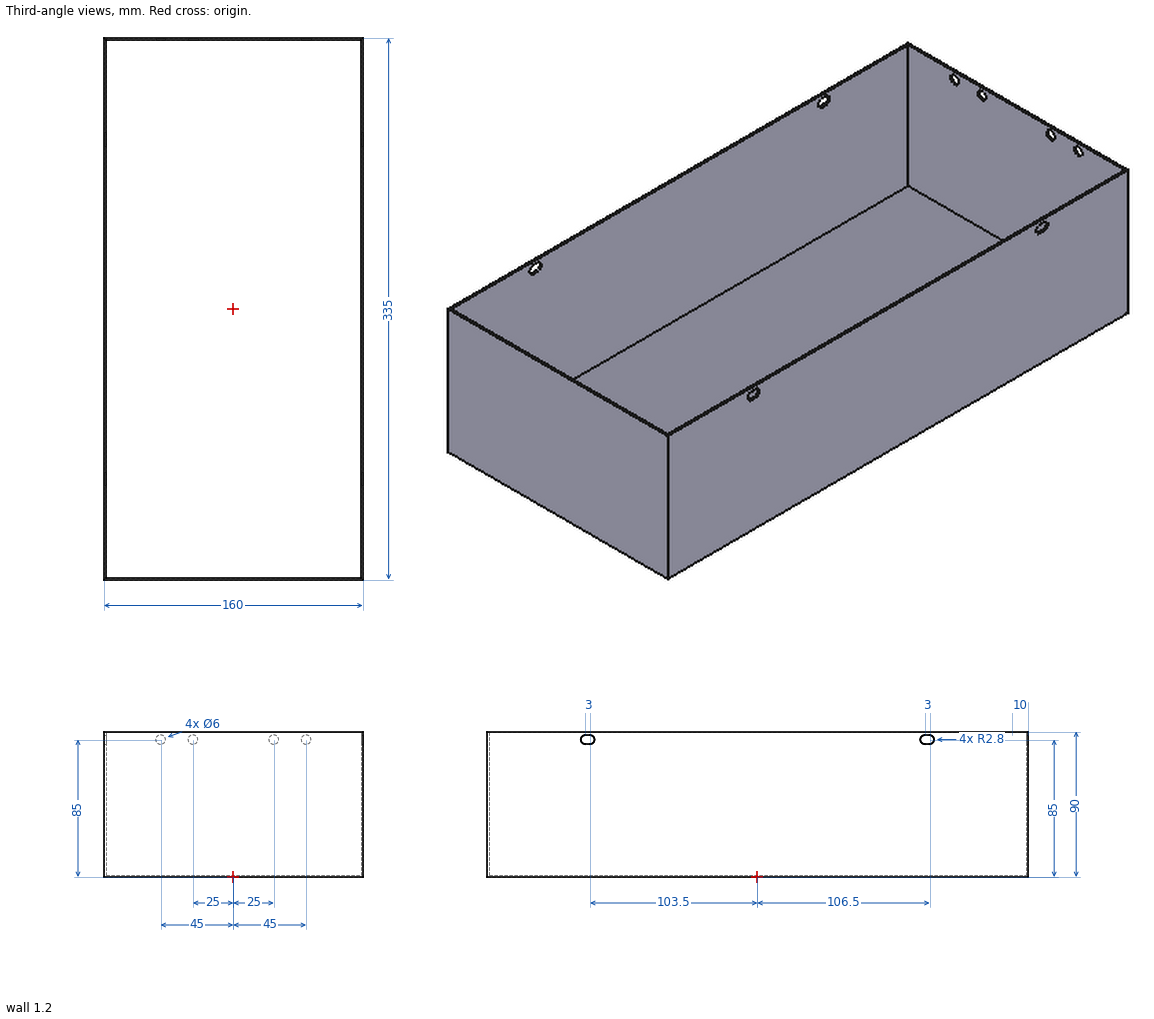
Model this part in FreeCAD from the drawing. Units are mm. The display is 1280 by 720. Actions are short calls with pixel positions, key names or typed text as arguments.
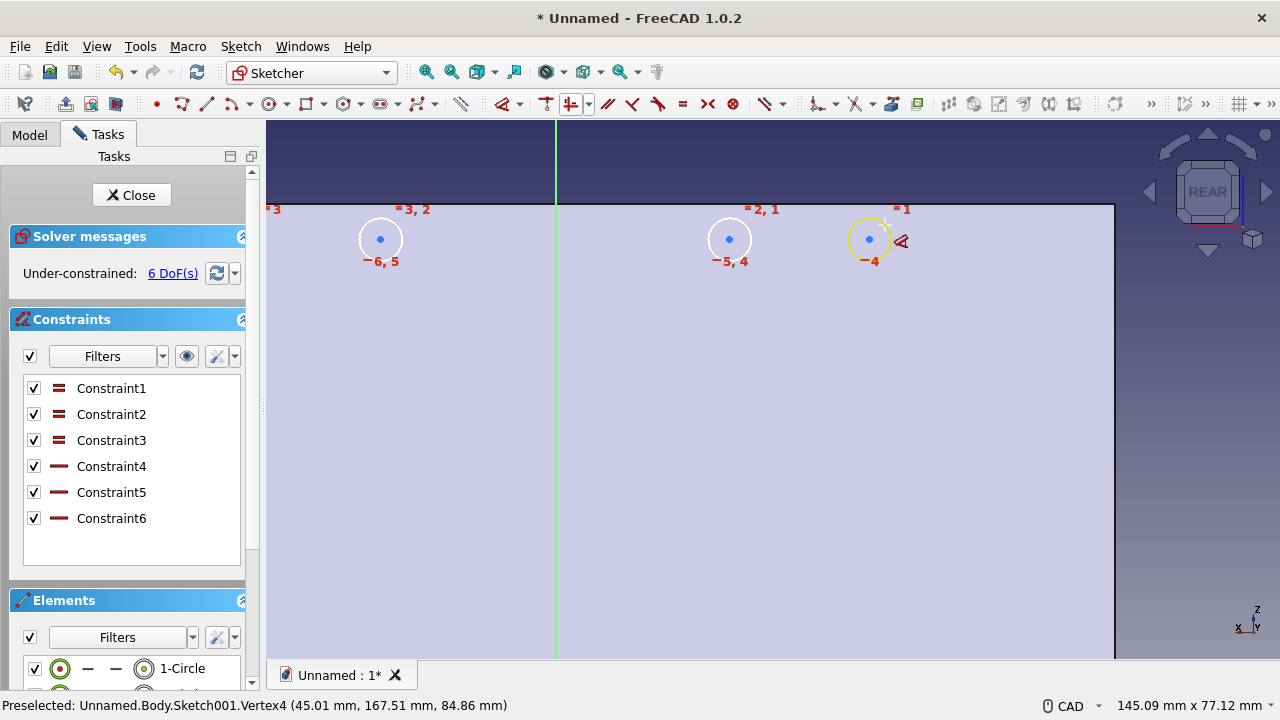
click(885, 225)
click(908, 203)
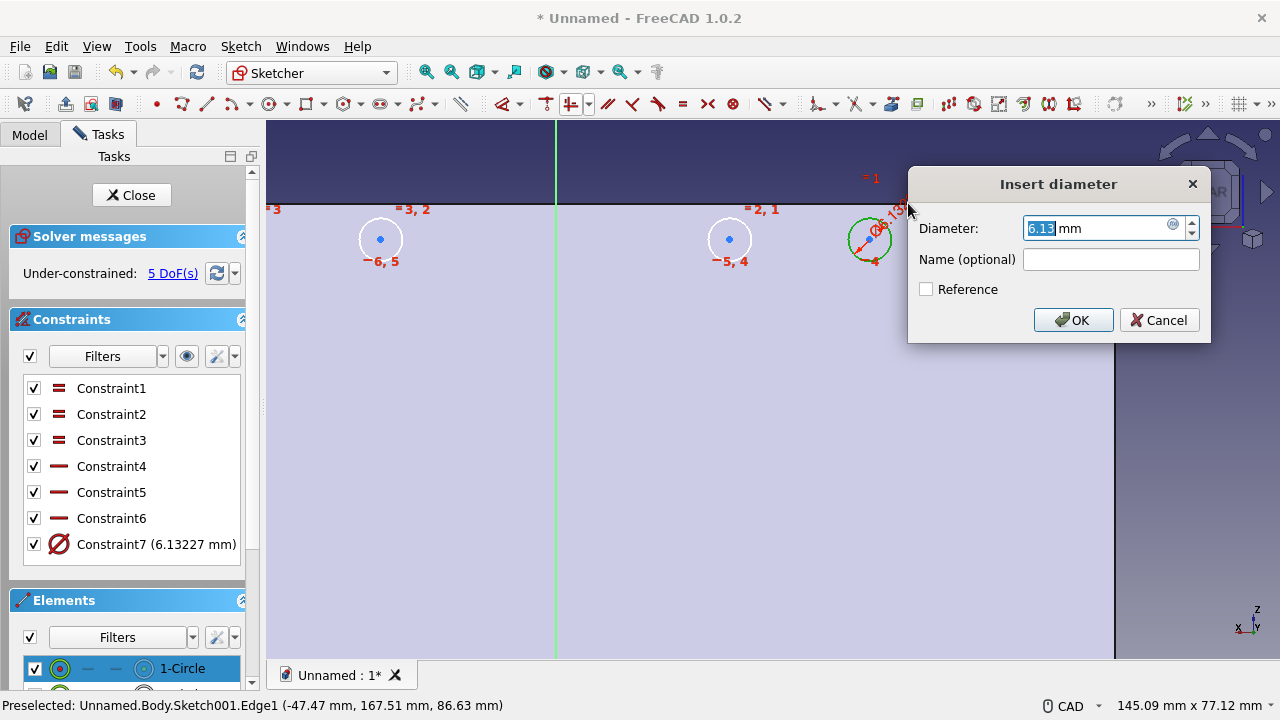
text(6)
key(Return)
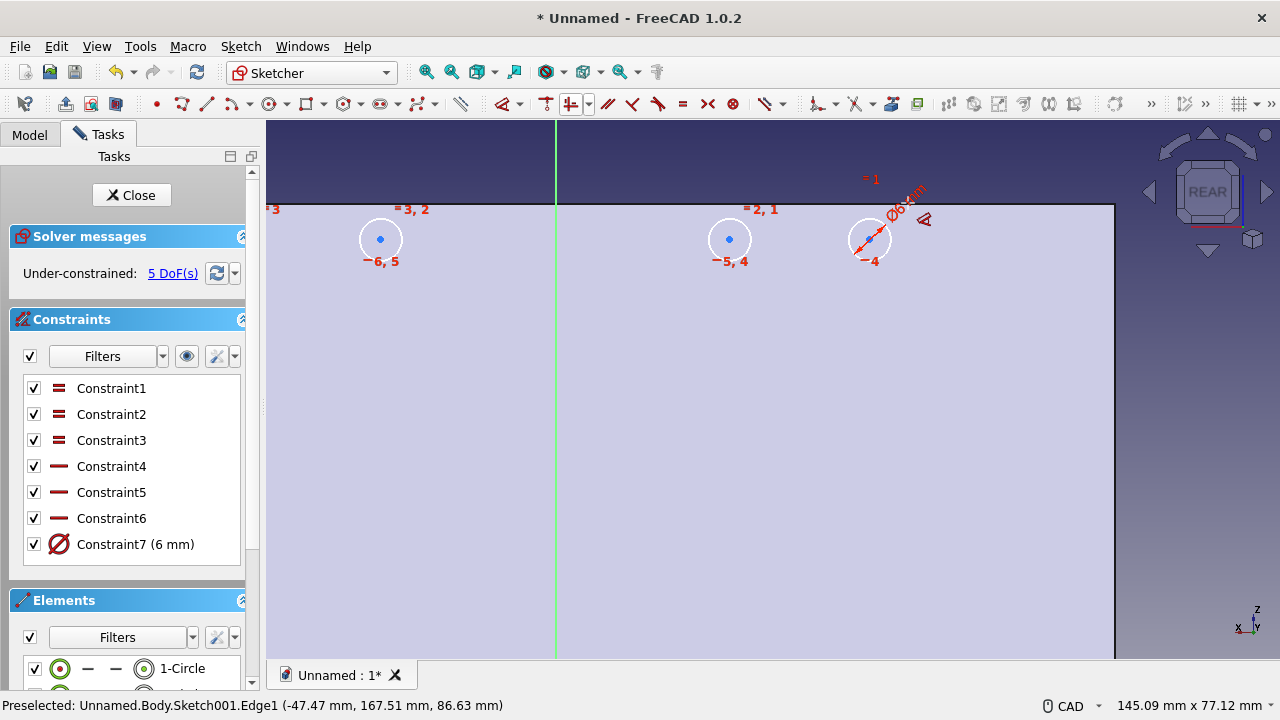
click(870, 240)
click(713, 206)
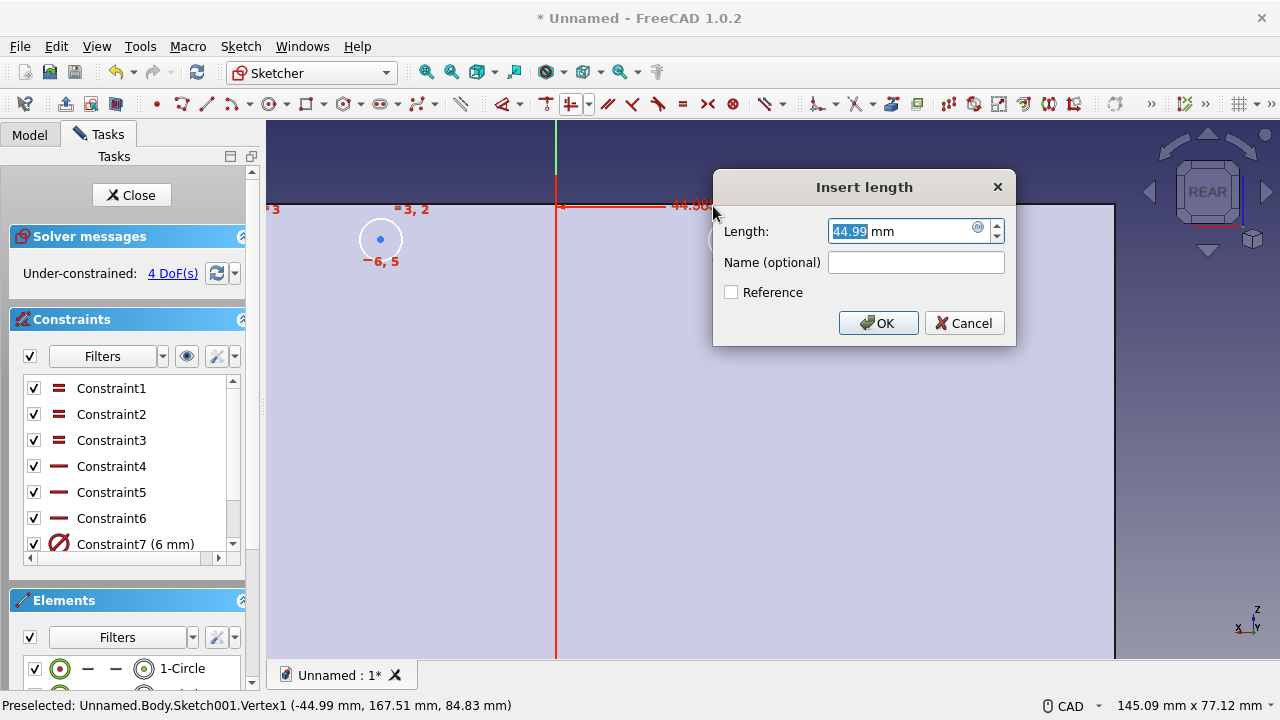
text(45)
key(Return)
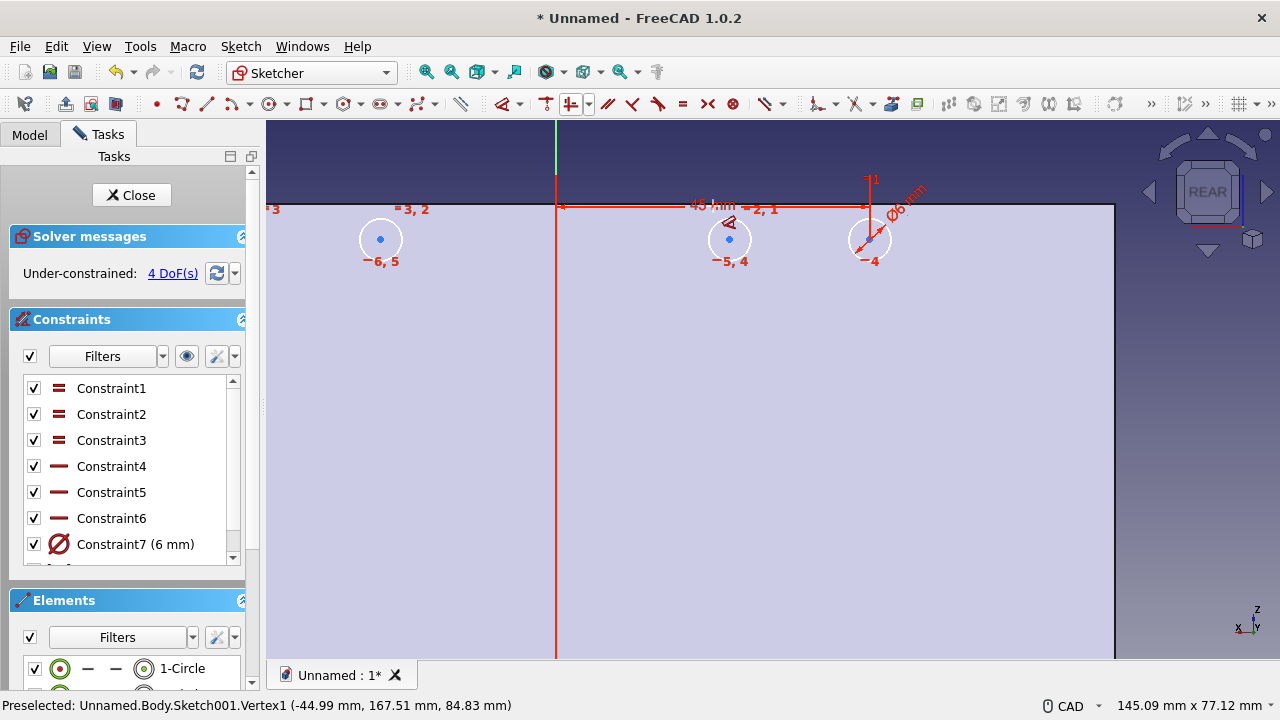
click(870, 240)
click(904, 435)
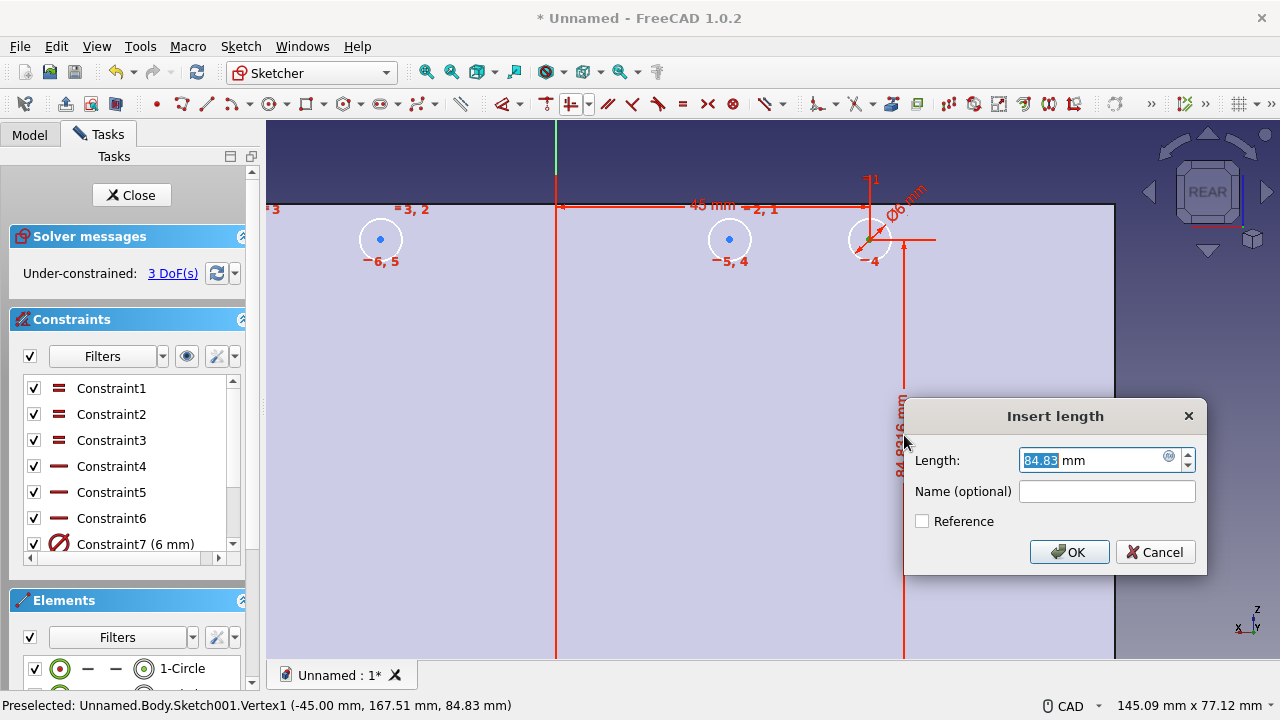
text(85)
key(Return)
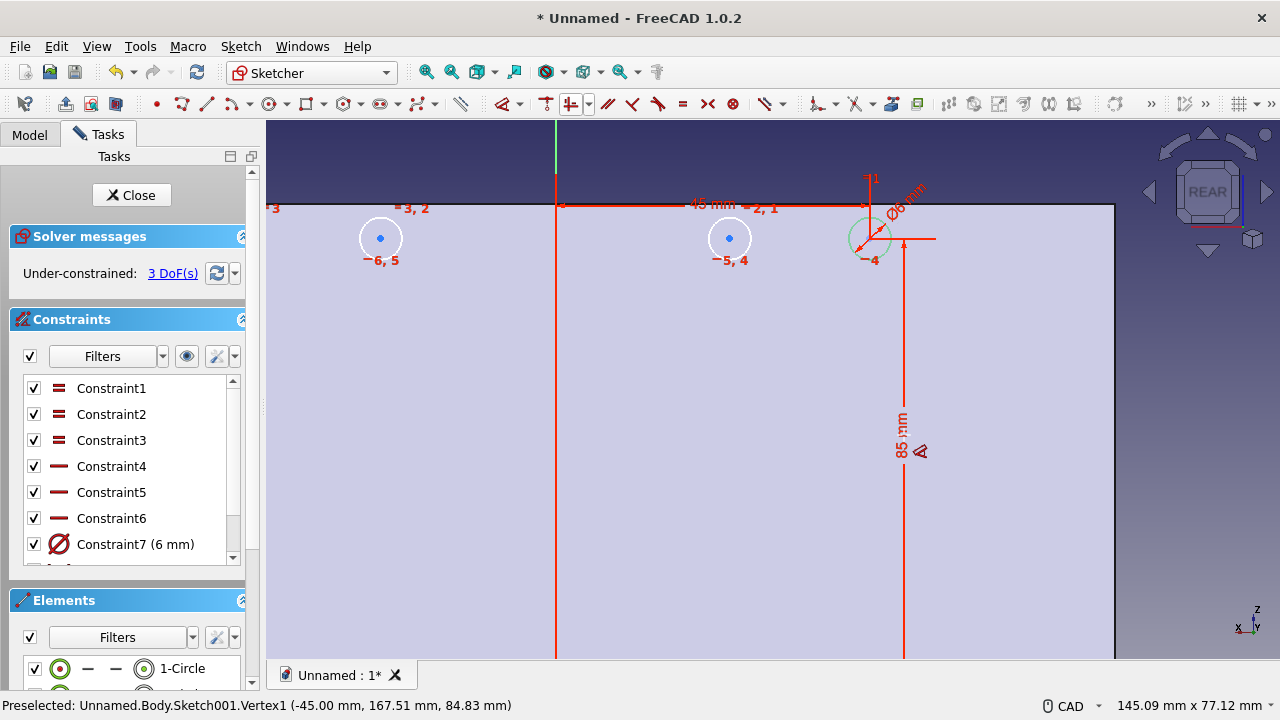
click(730, 239)
click(643, 205)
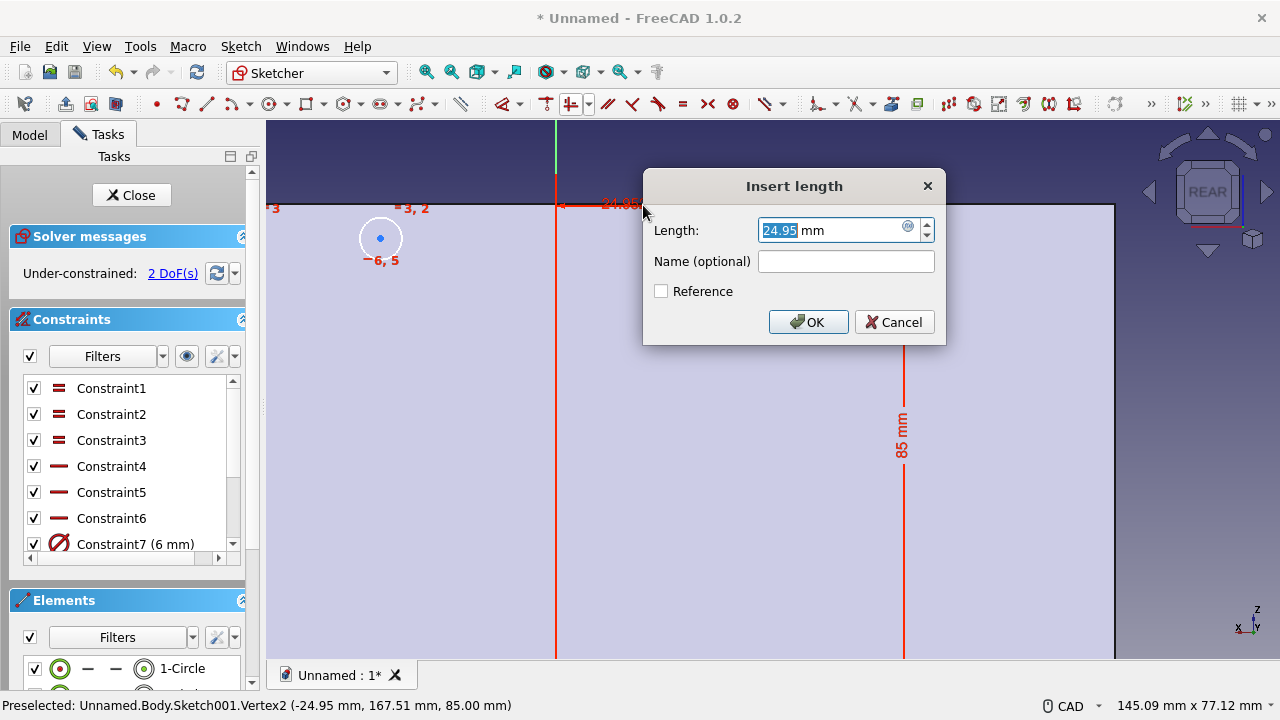
text(25)
key(Return)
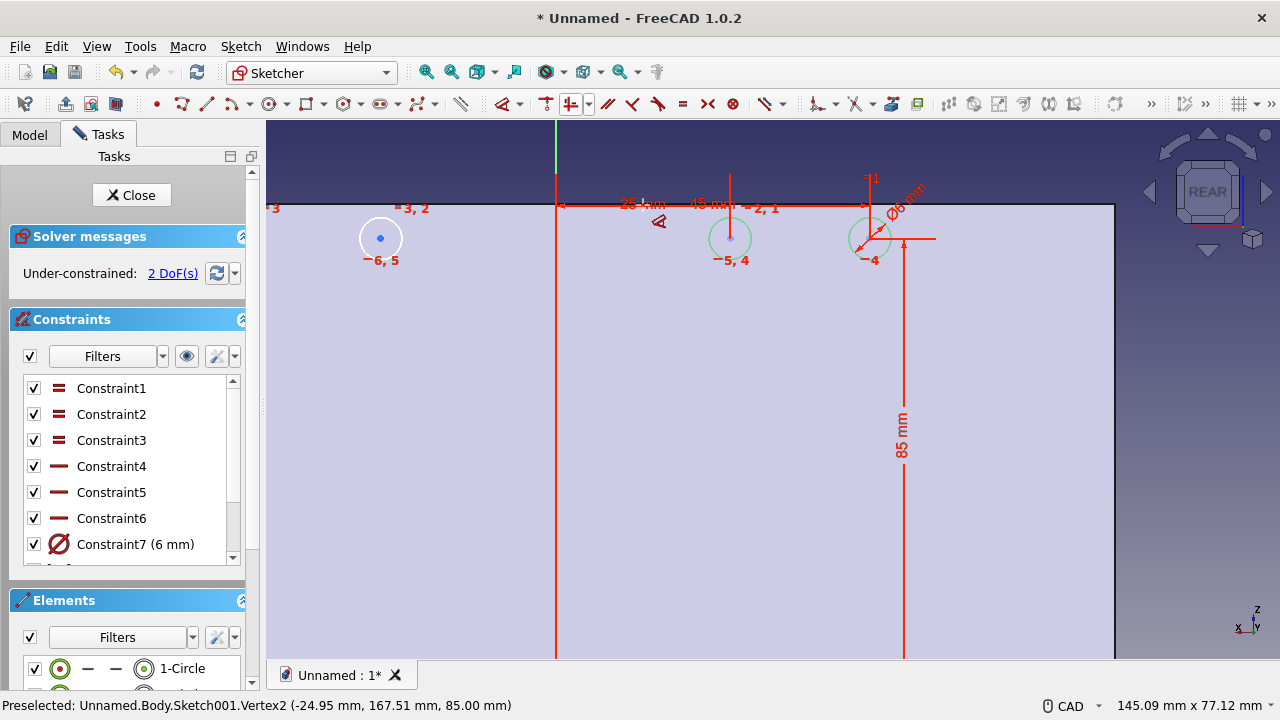
click(381, 239)
click(468, 205)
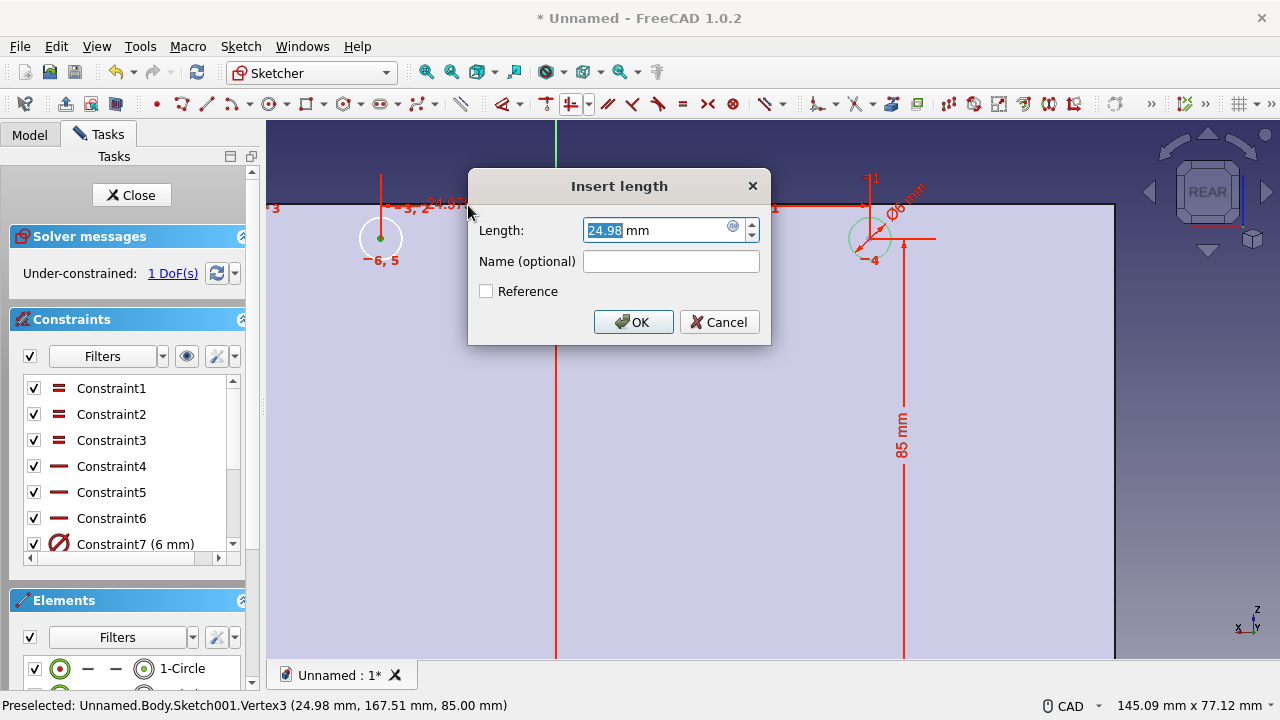
text(25)
key(Return)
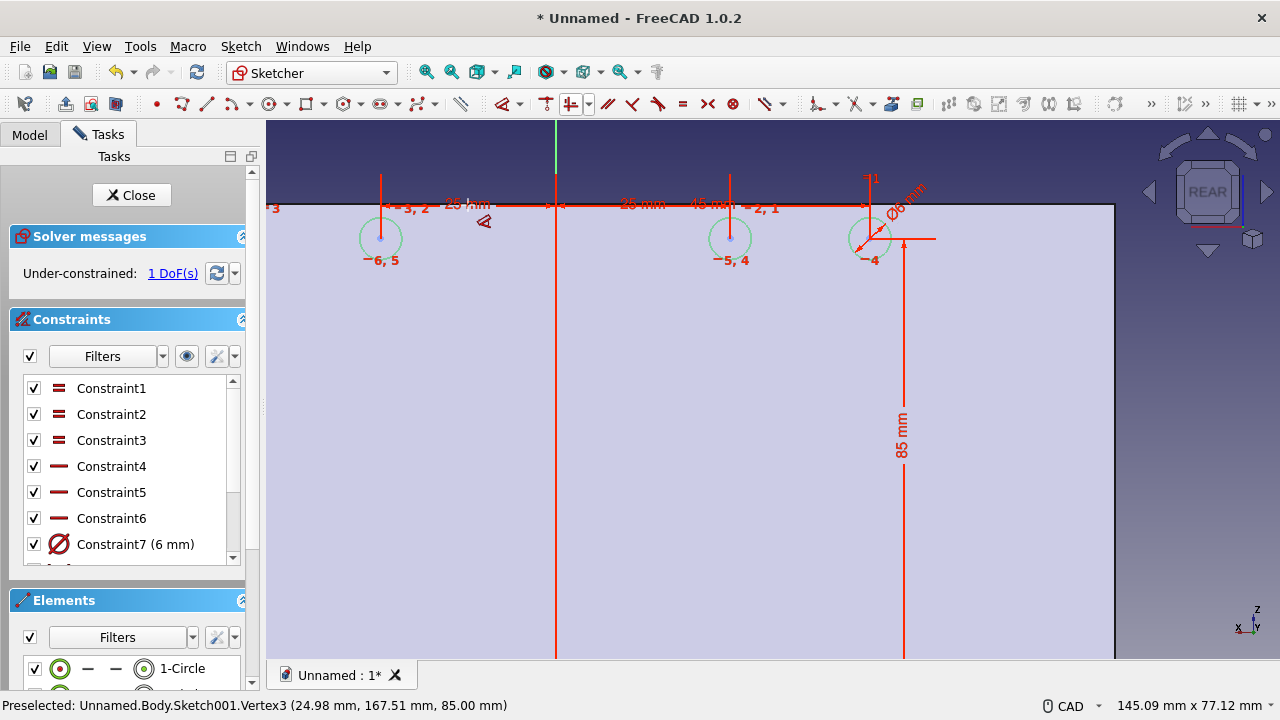
scroll(886, 224, down, 3)